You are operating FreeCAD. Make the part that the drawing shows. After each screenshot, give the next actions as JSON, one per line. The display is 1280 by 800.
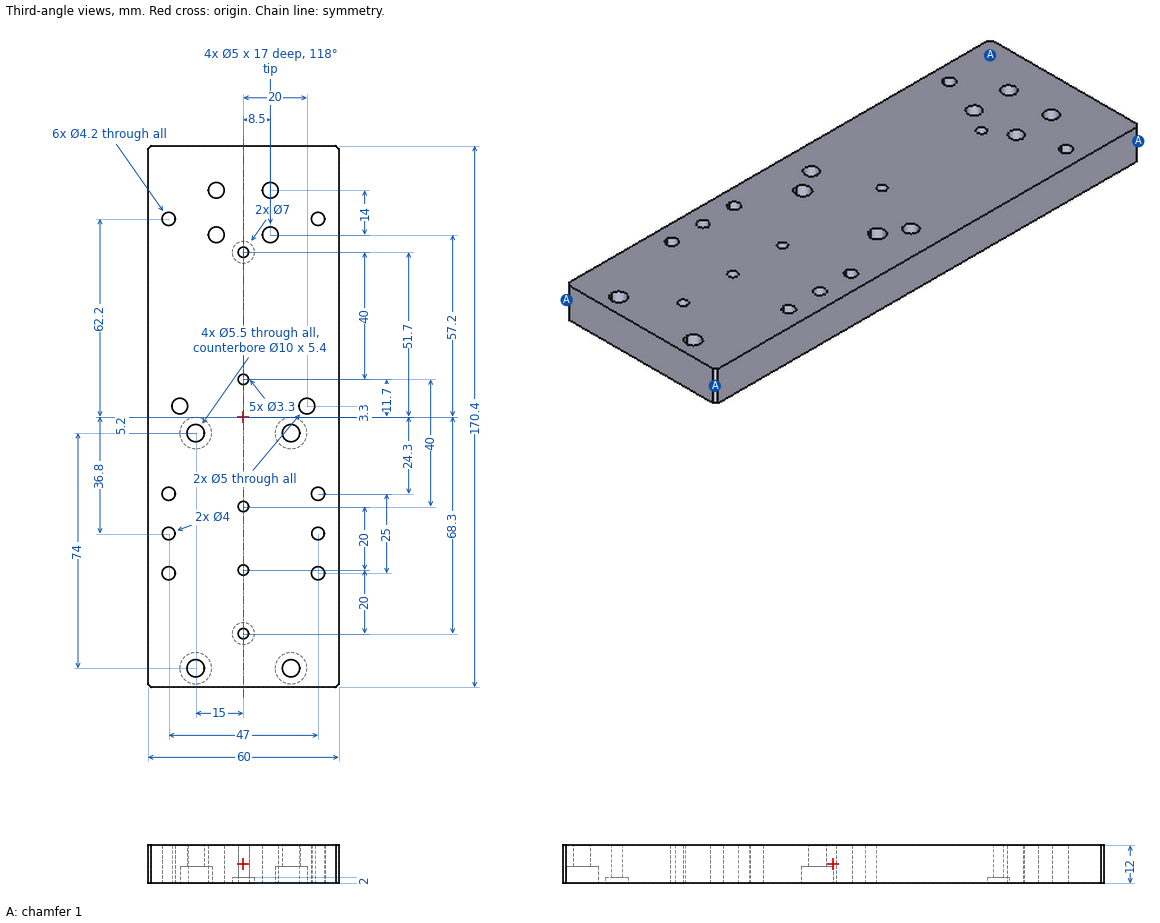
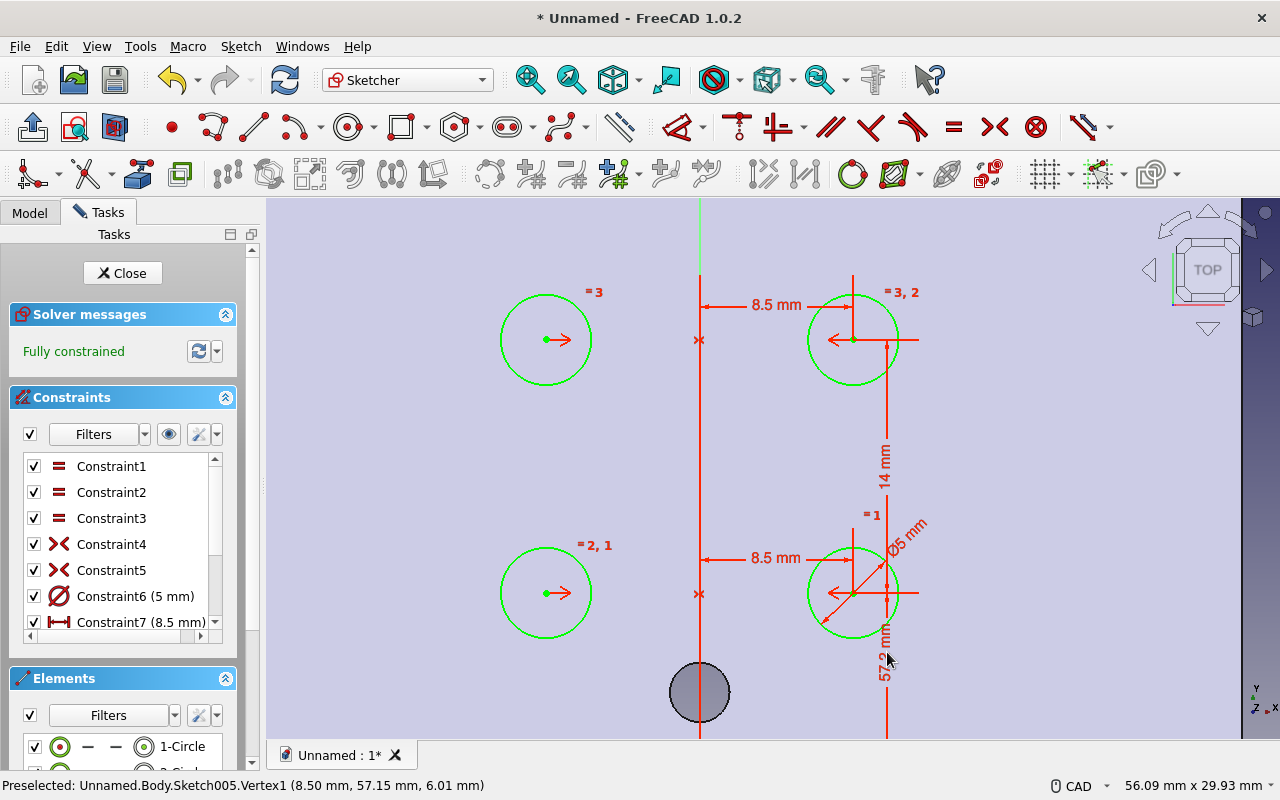
{"action": "left_click", "coordinate": [123, 273]}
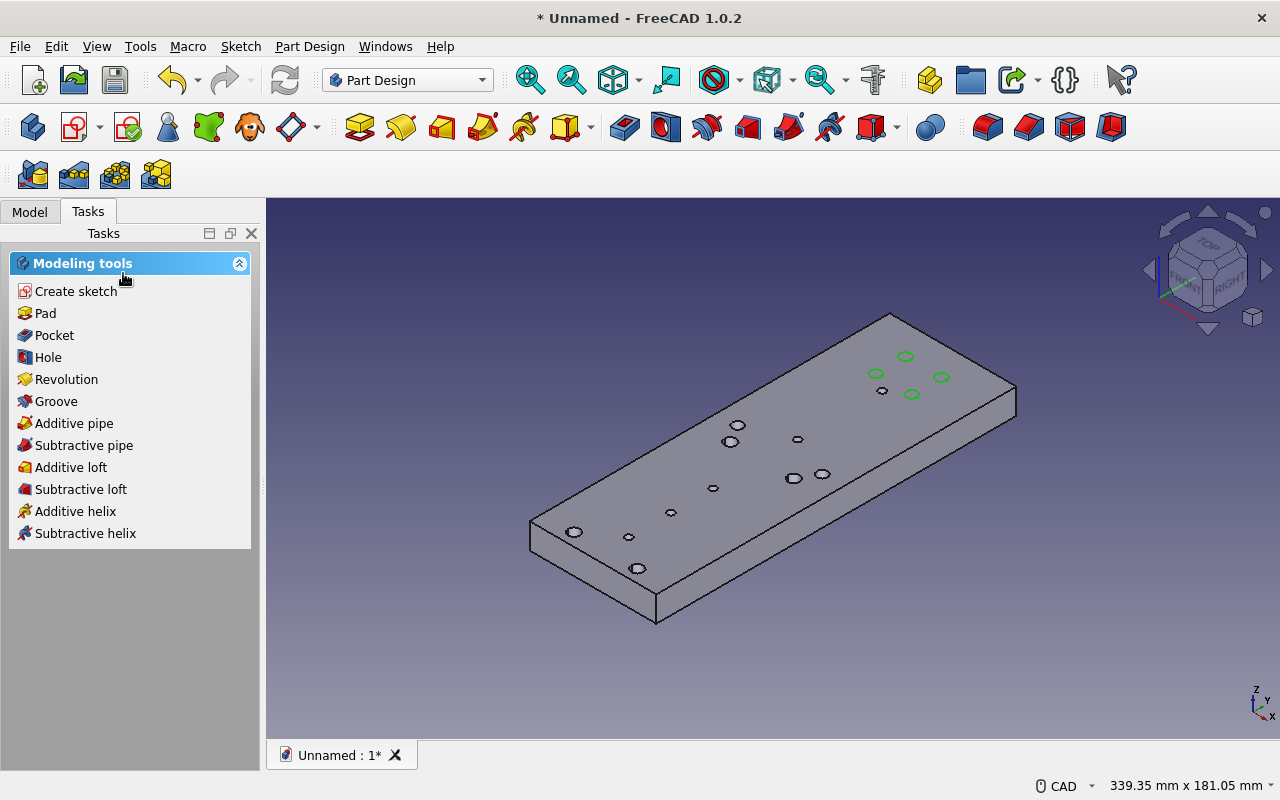
{"action": "left_click", "coordinate": [666, 128]}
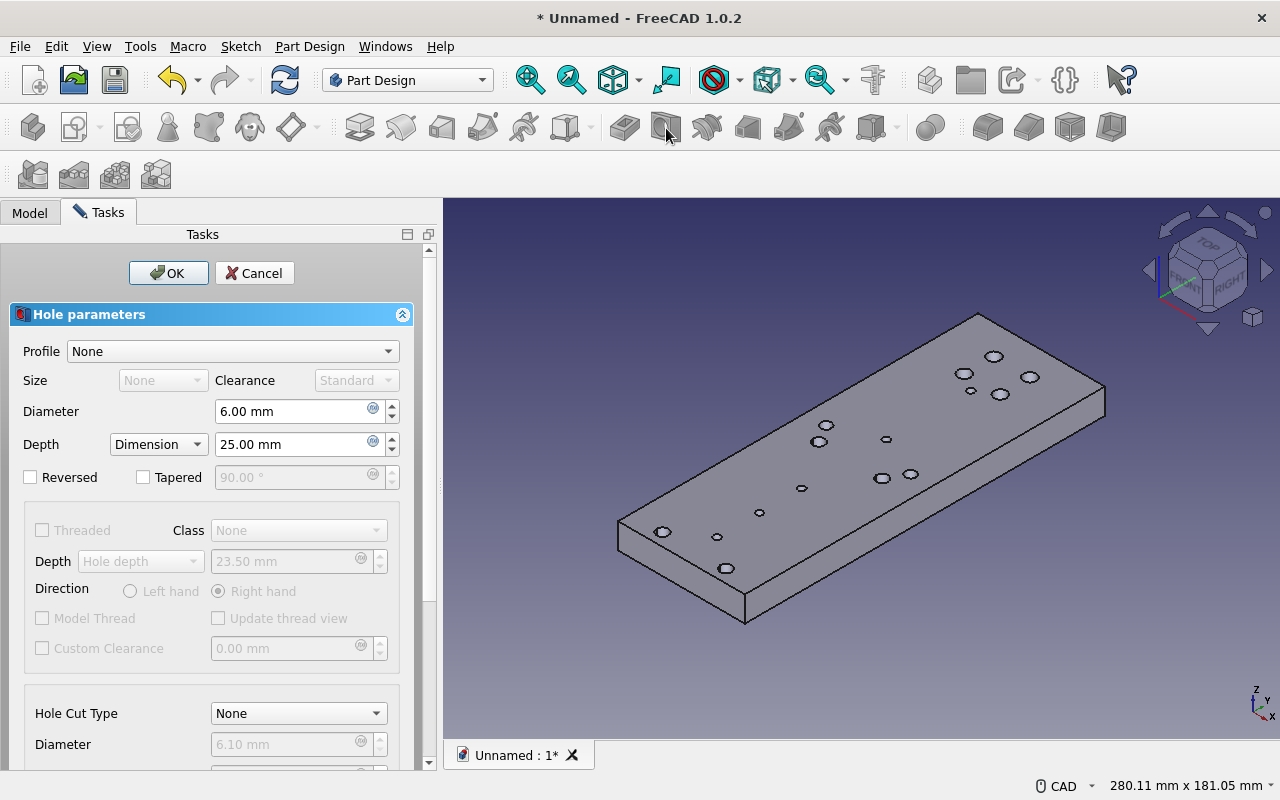
{"action": "triple_click", "coordinate": [300, 412]}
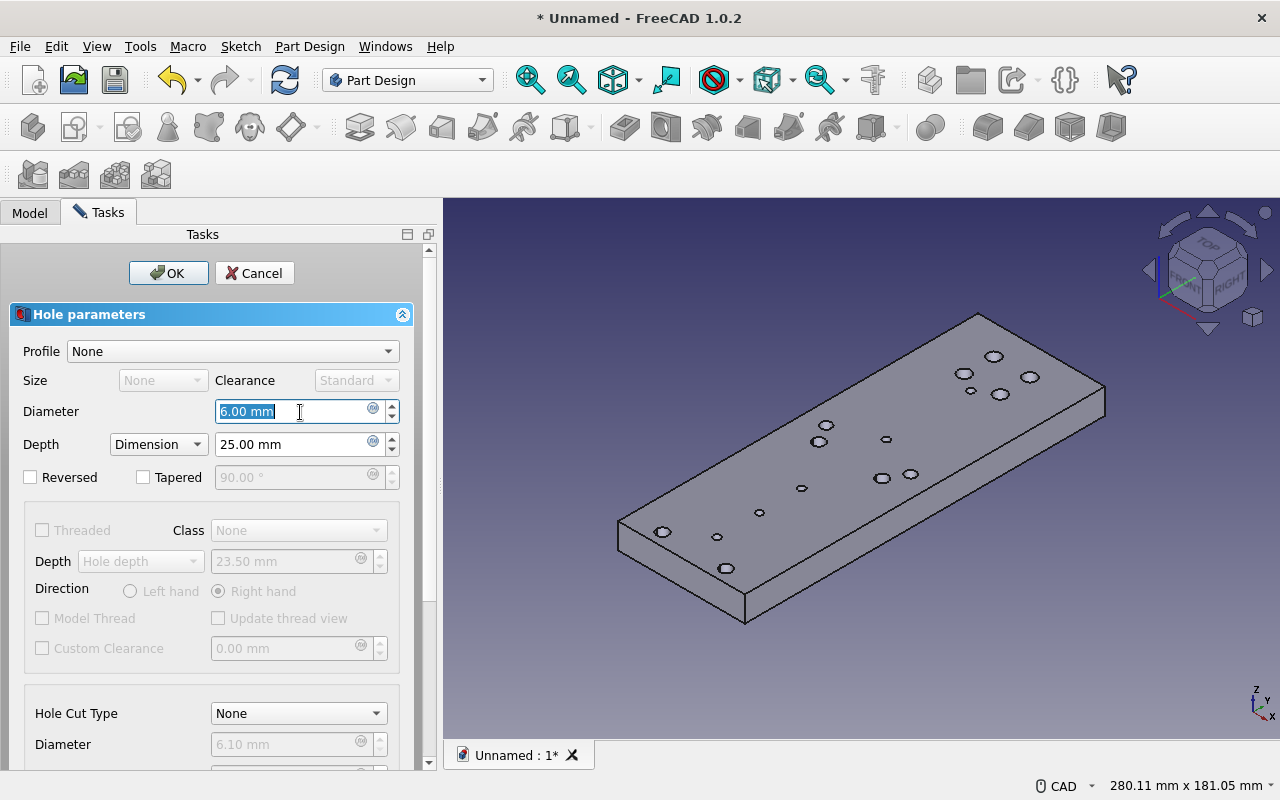
{"action": "type", "text": "5"}
{"action": "key", "text": "Tab"}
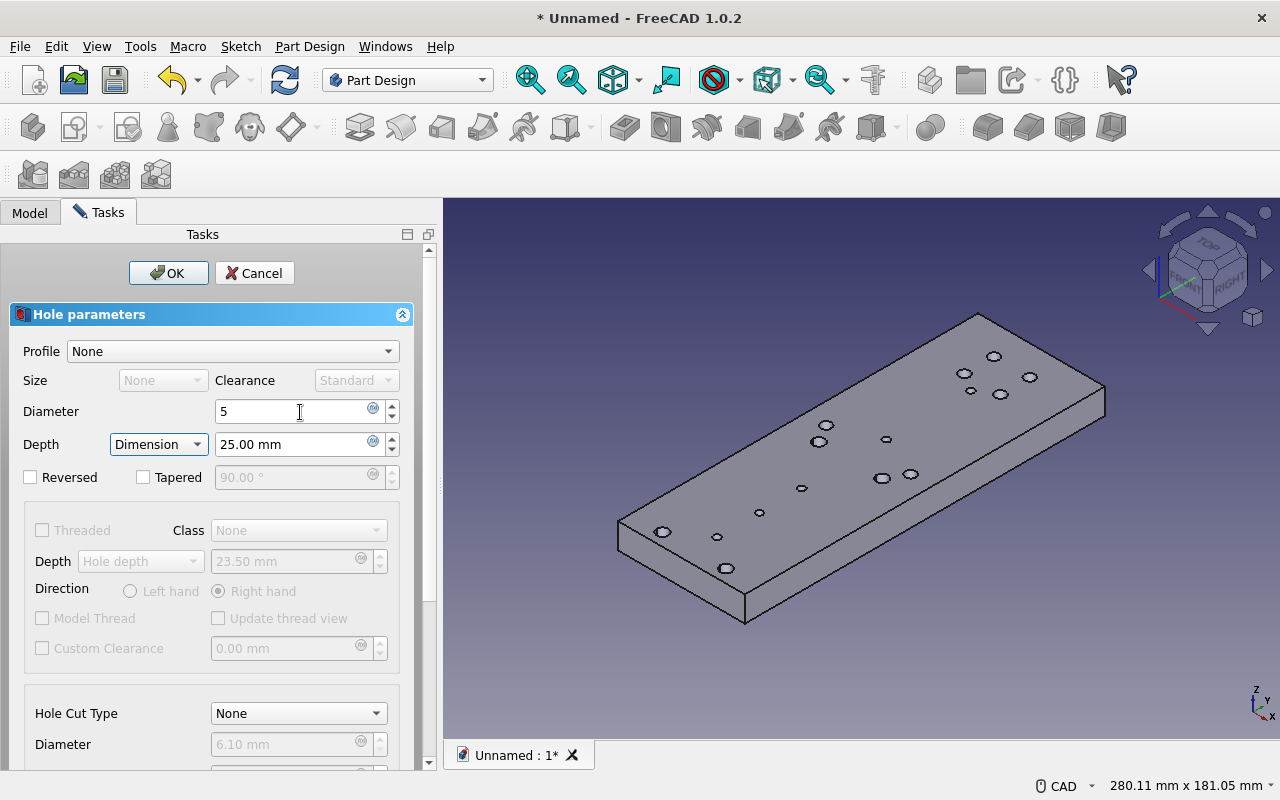
{"action": "triple_click", "coordinate": [300, 444]}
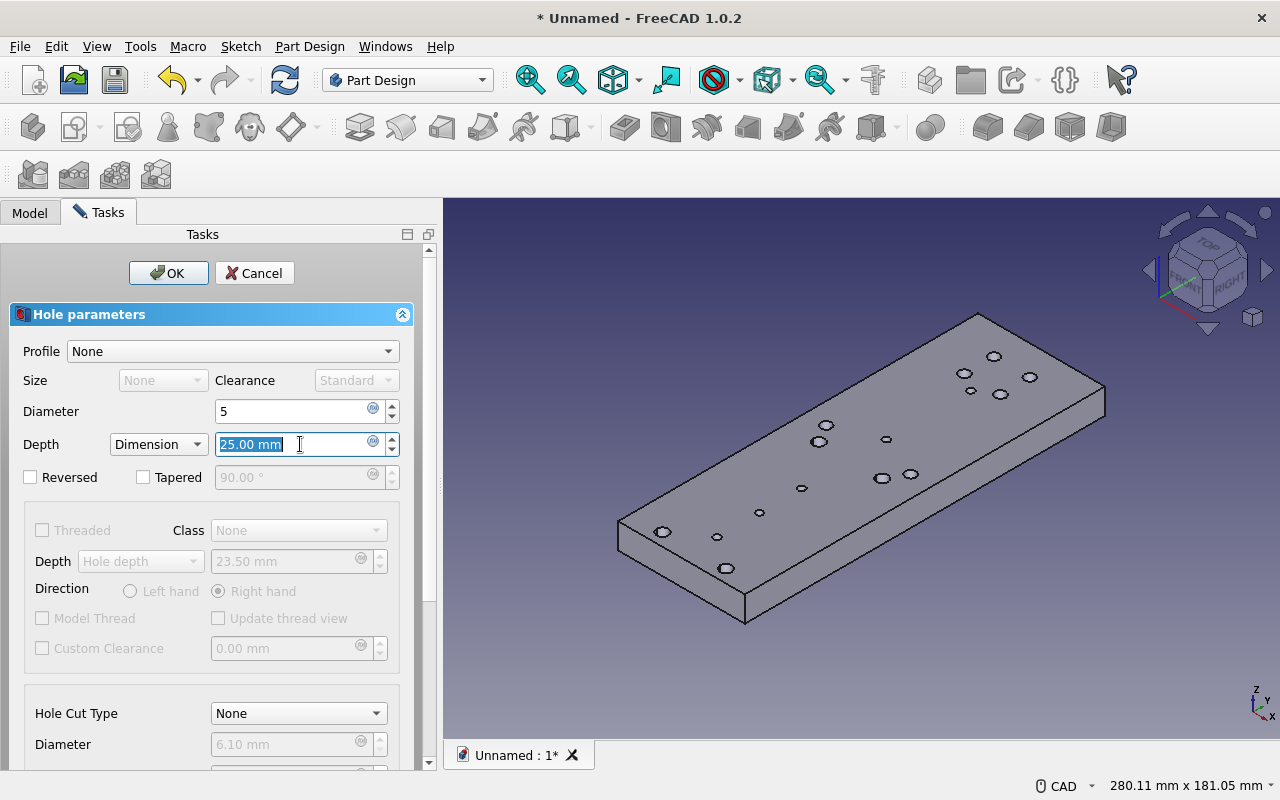
{"action": "type", "text": "17"}
{"action": "key", "text": "Tab"}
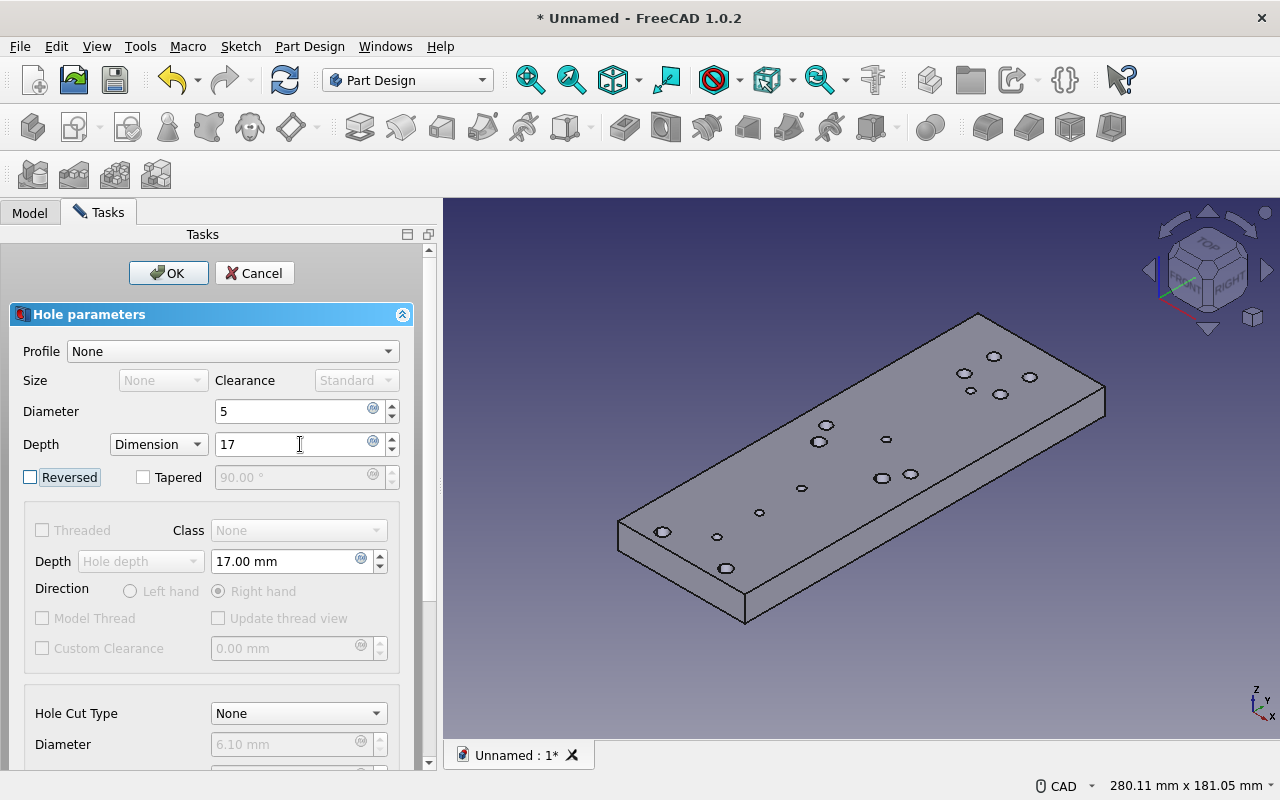
{"action": "left_click", "coordinate": [169, 273]}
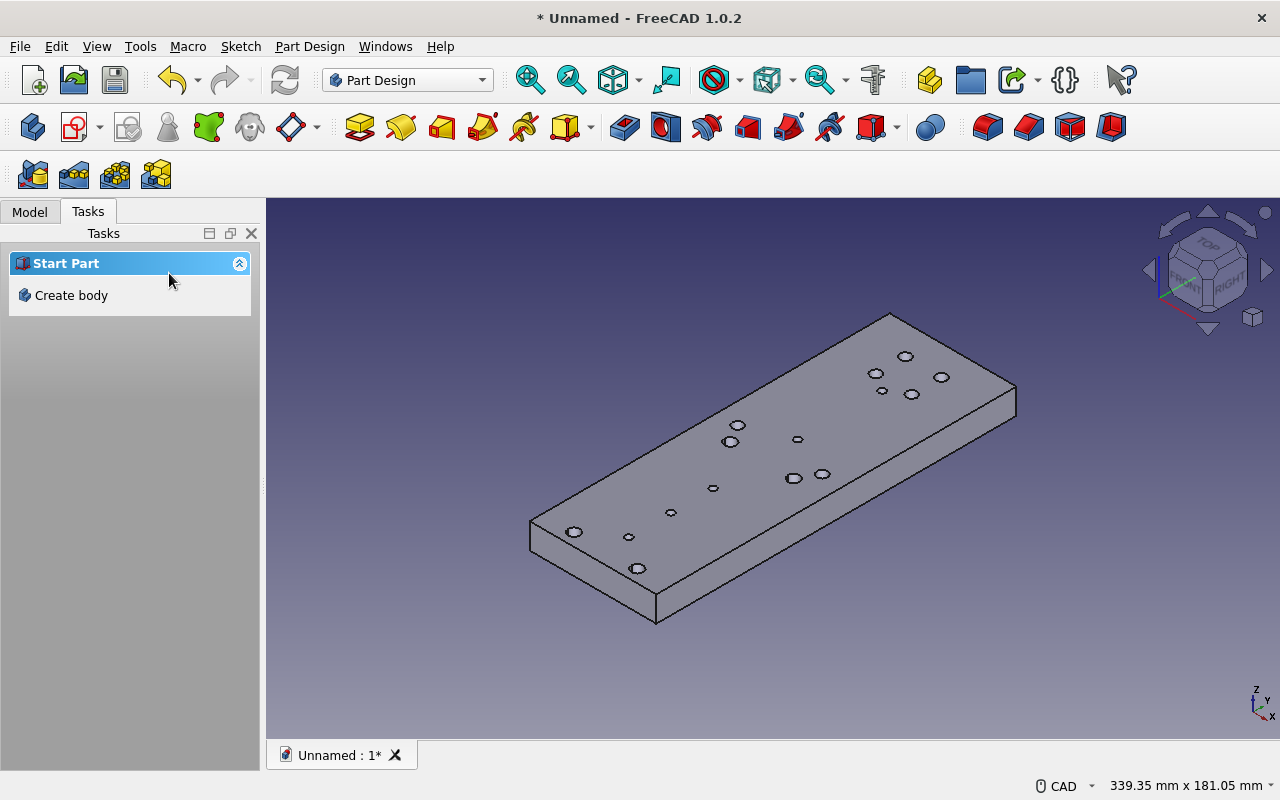
{"action": "left_click", "coordinate": [656, 608]}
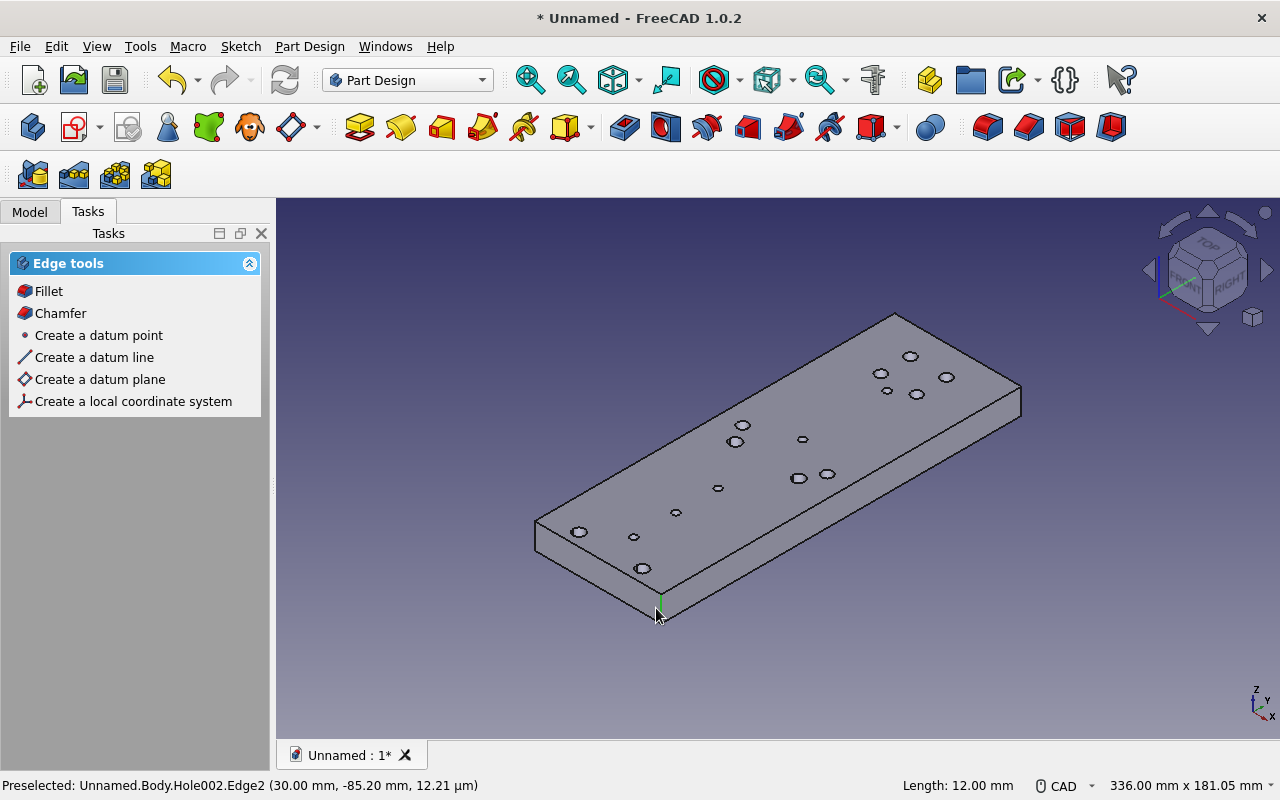
{"action": "key", "text": "2"}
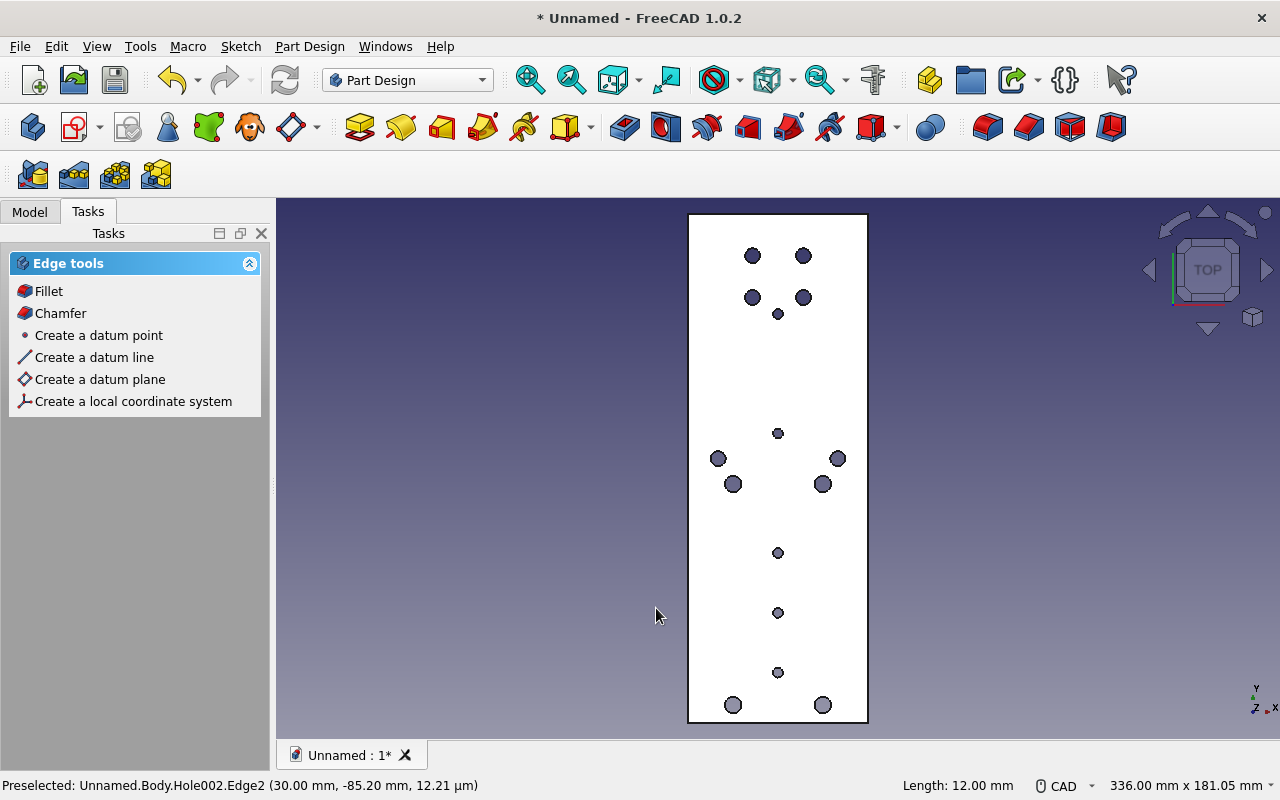
{"action": "key", "text": "0"}